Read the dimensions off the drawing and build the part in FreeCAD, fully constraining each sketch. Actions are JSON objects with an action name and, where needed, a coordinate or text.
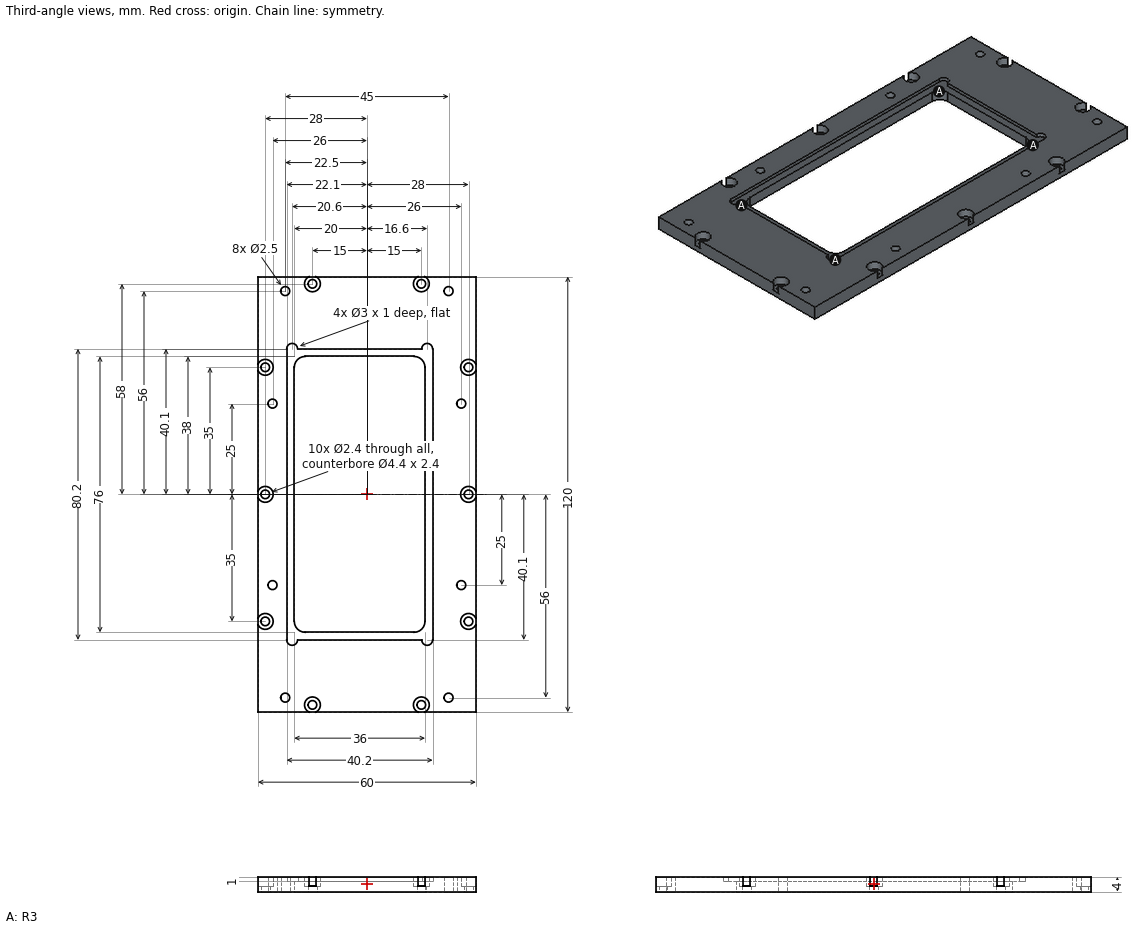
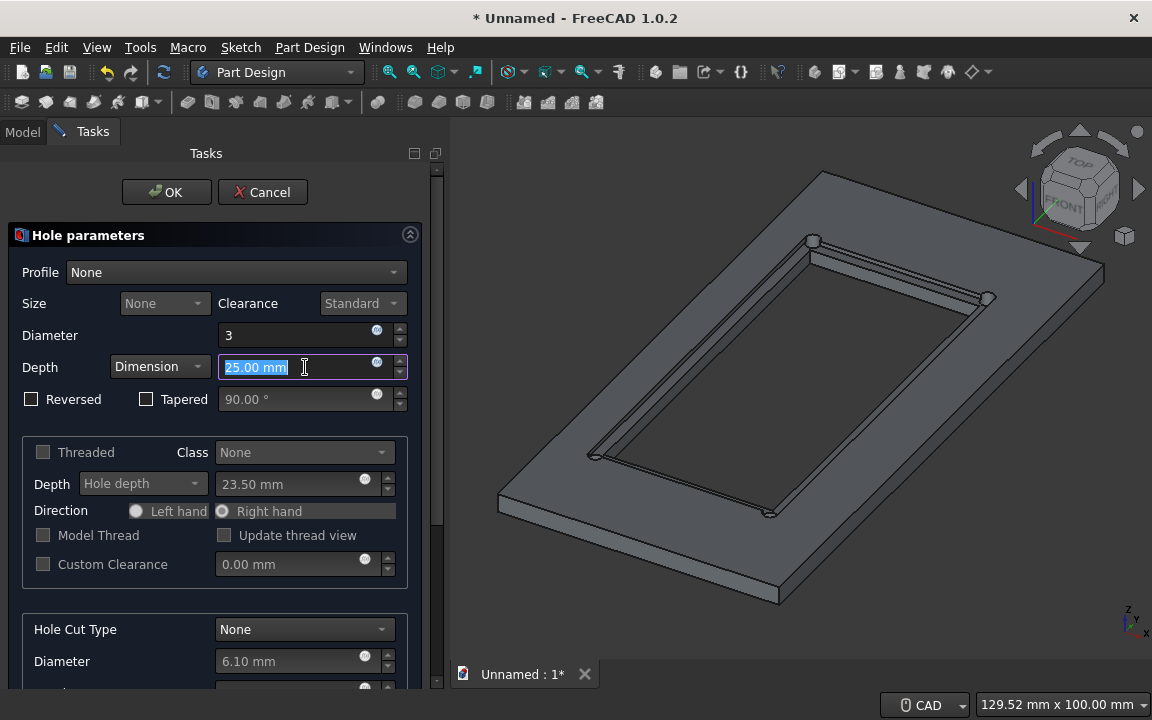
{"action": "type", "text": "1"}
{"action": "key", "text": "Tab"}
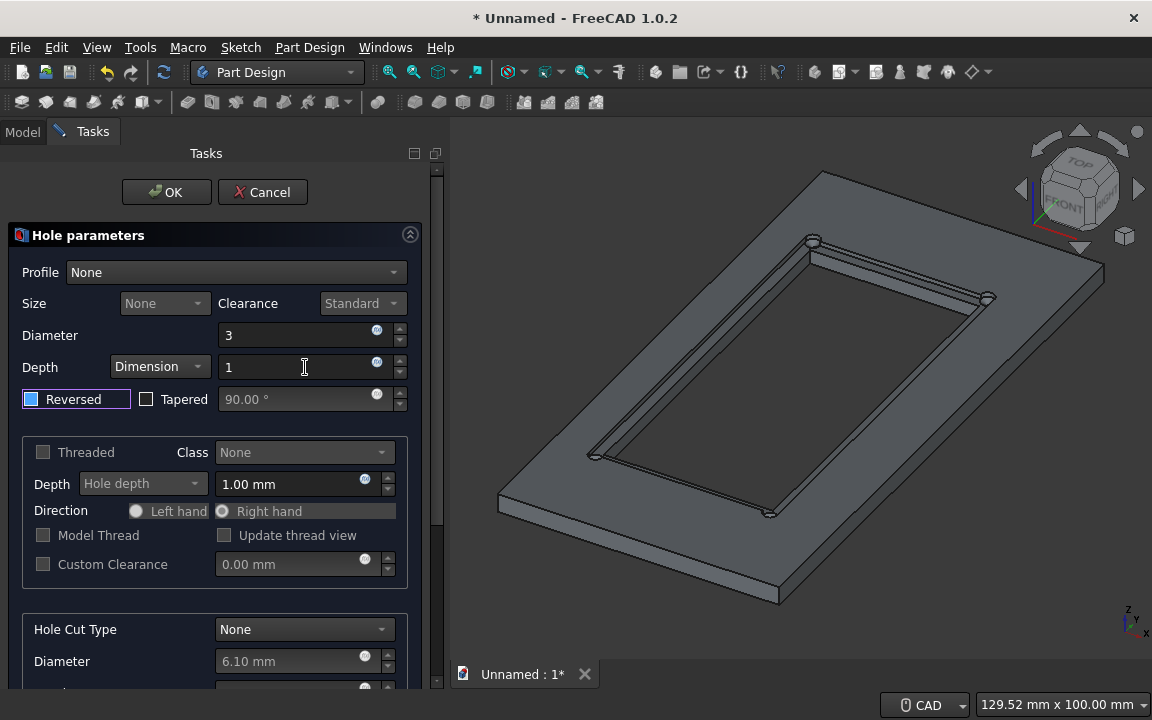
{"action": "scroll", "coordinate": [437, 426], "scroll_direction": "down", "scroll_amount": 4}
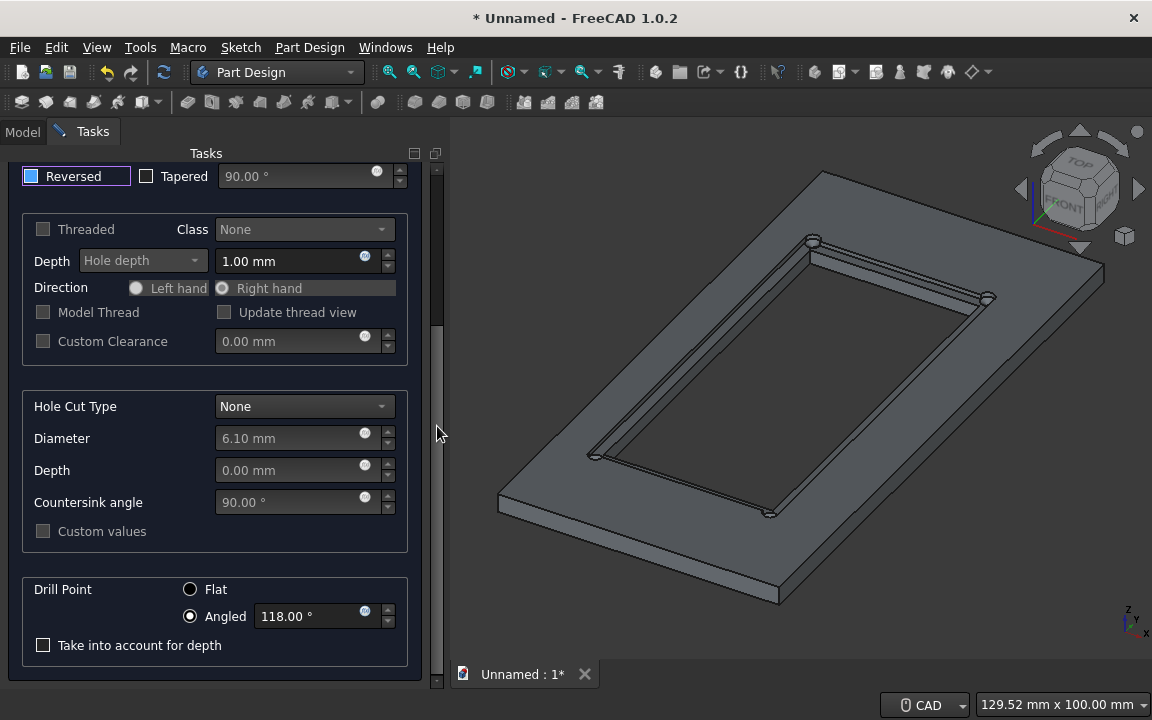
{"action": "left_click", "coordinate": [191, 589]}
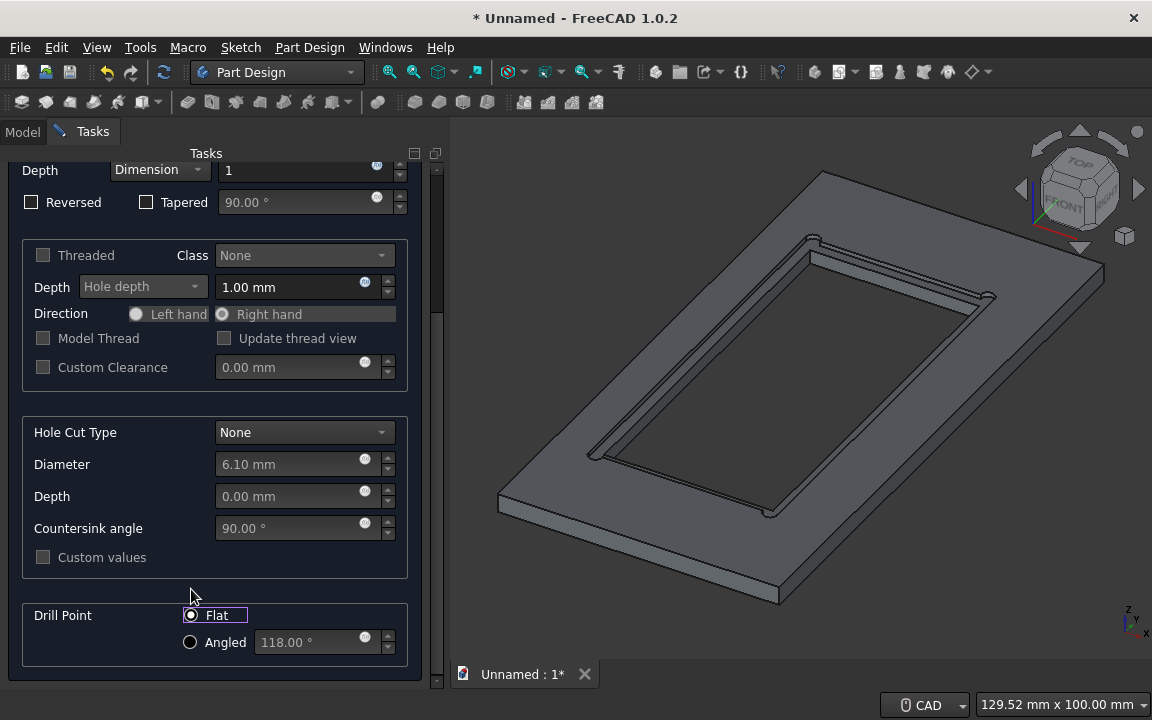
{"action": "scroll", "coordinate": [437, 426], "scroll_direction": "up", "scroll_amount": 5}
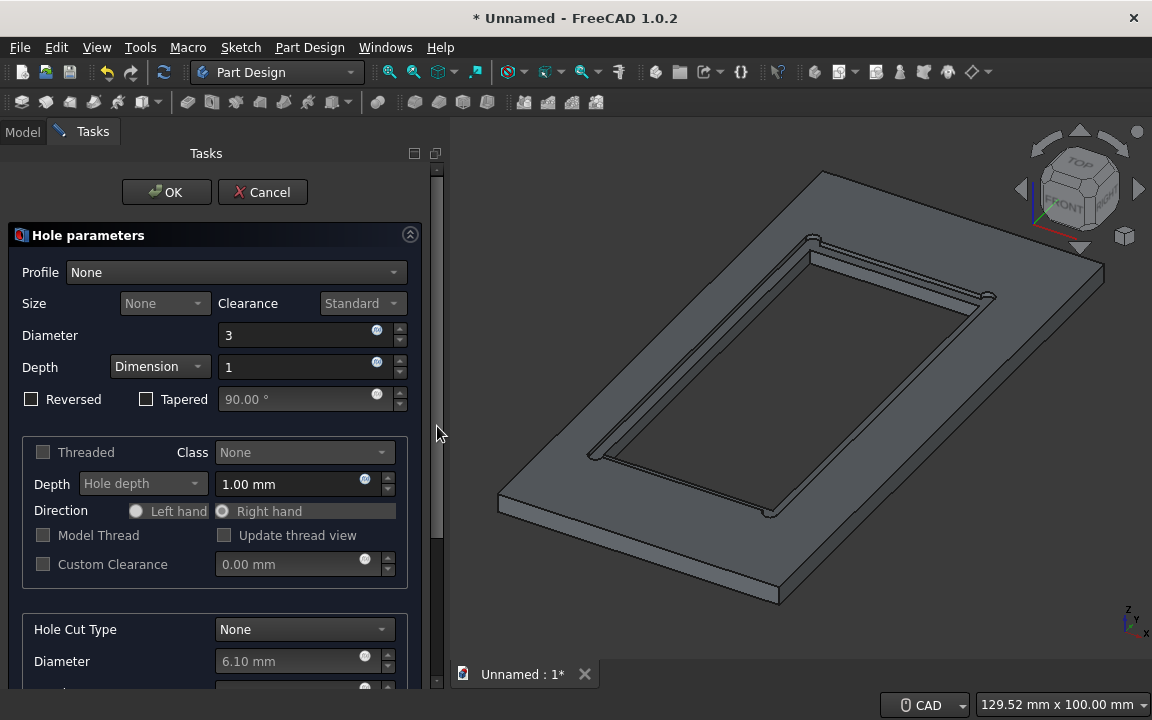
{"action": "left_click", "coordinate": [167, 192]}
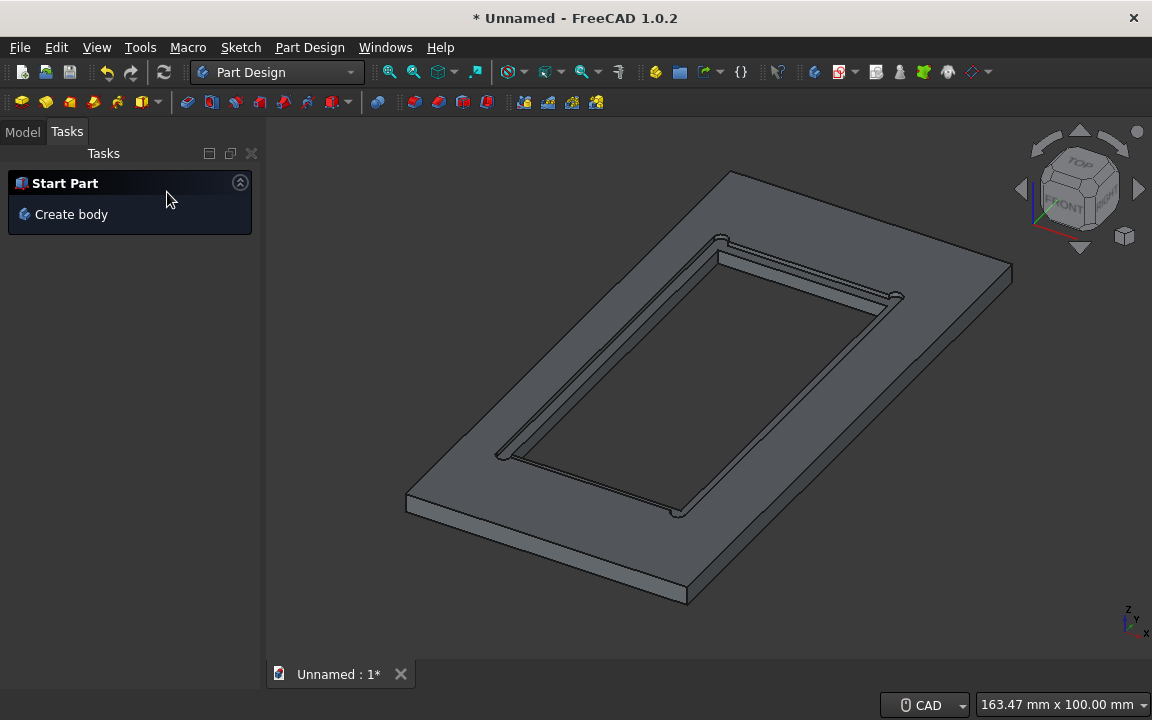
{"action": "scroll", "coordinate": [512, 460], "scroll_direction": "up", "scroll_amount": 5}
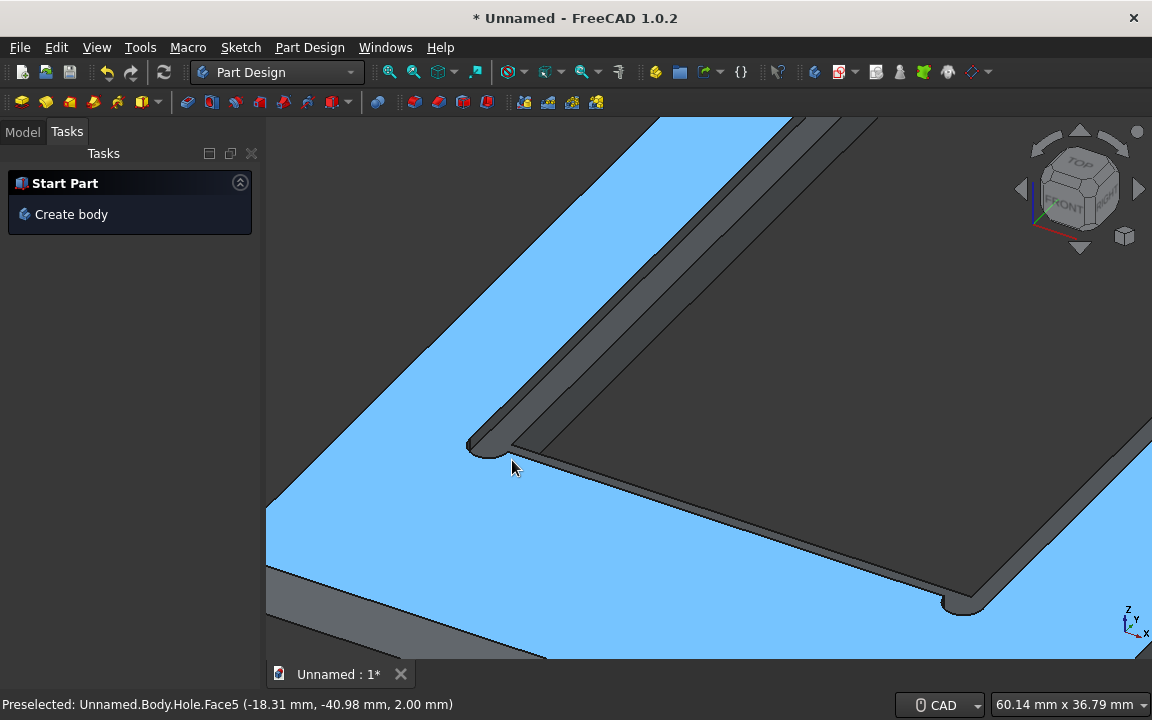
{"action": "key", "text": "v f"}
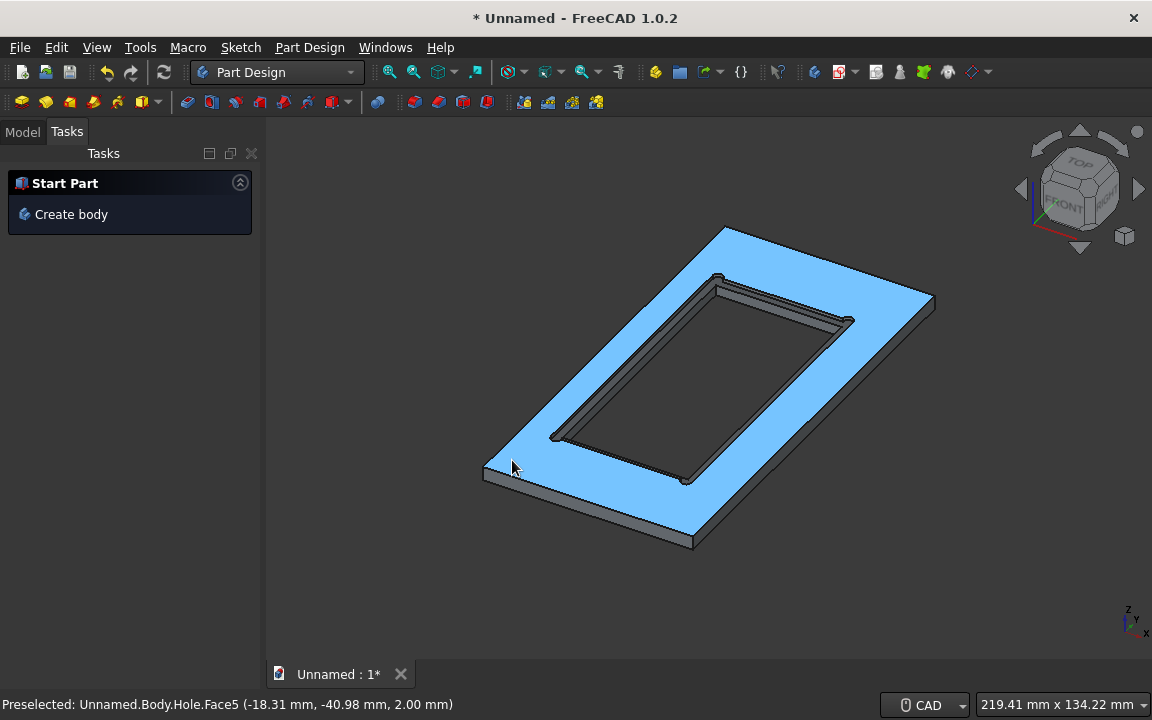
{"action": "key", "text": "0"}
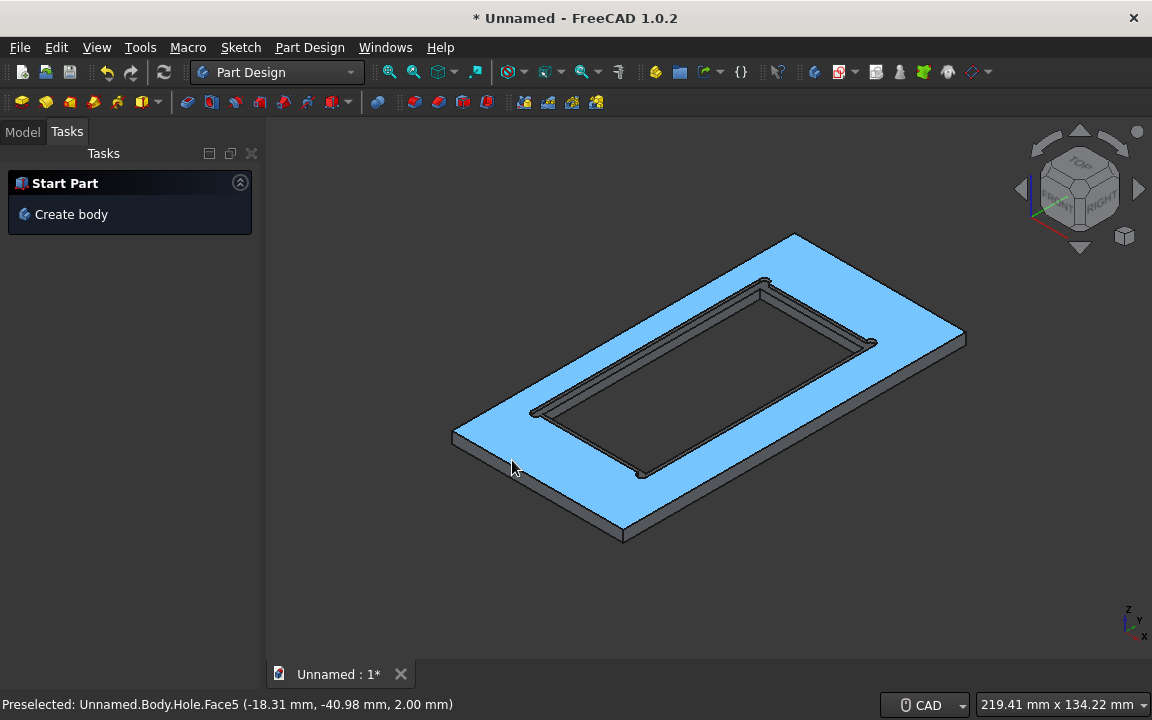
{"action": "scroll", "coordinate": [543, 418], "scroll_direction": "up", "scroll_amount": 6}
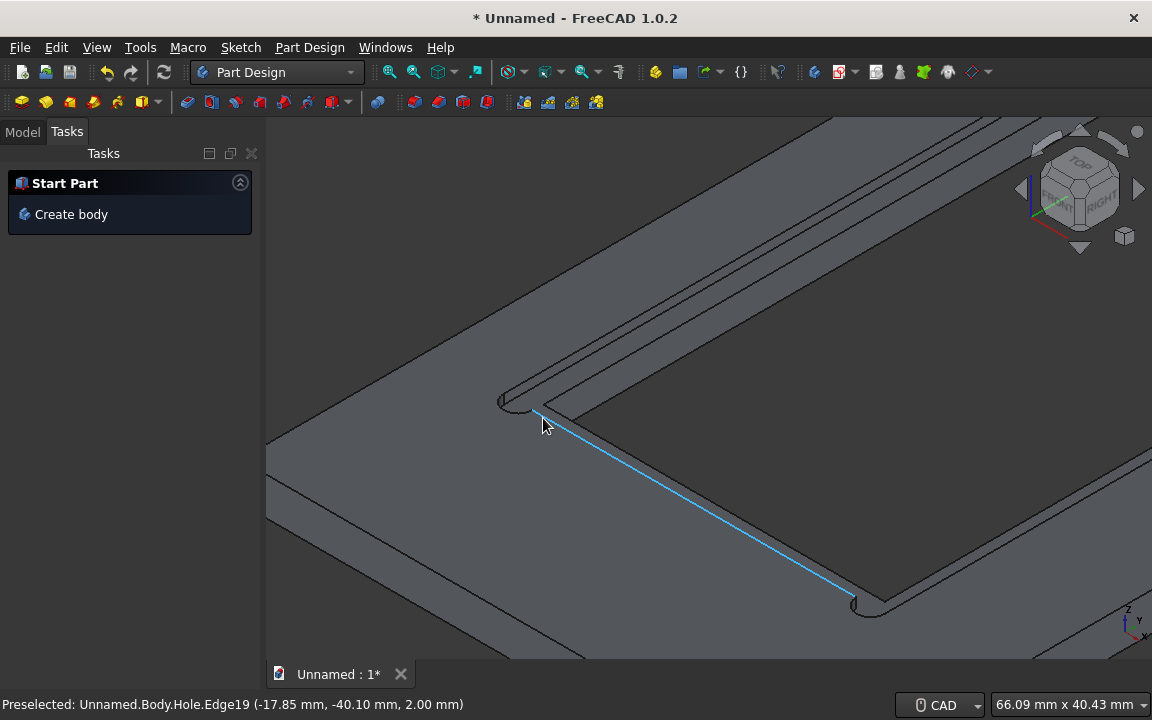
{"action": "left_click", "coordinate": [390, 72]}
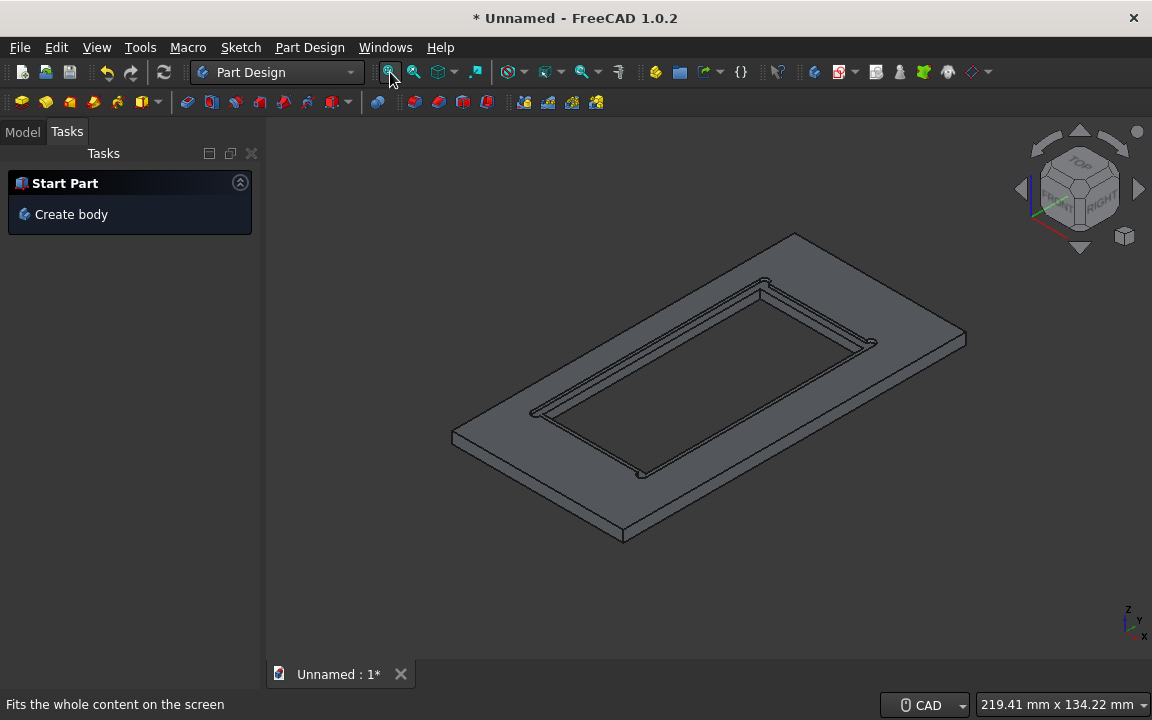
{"action": "key", "text": "2"}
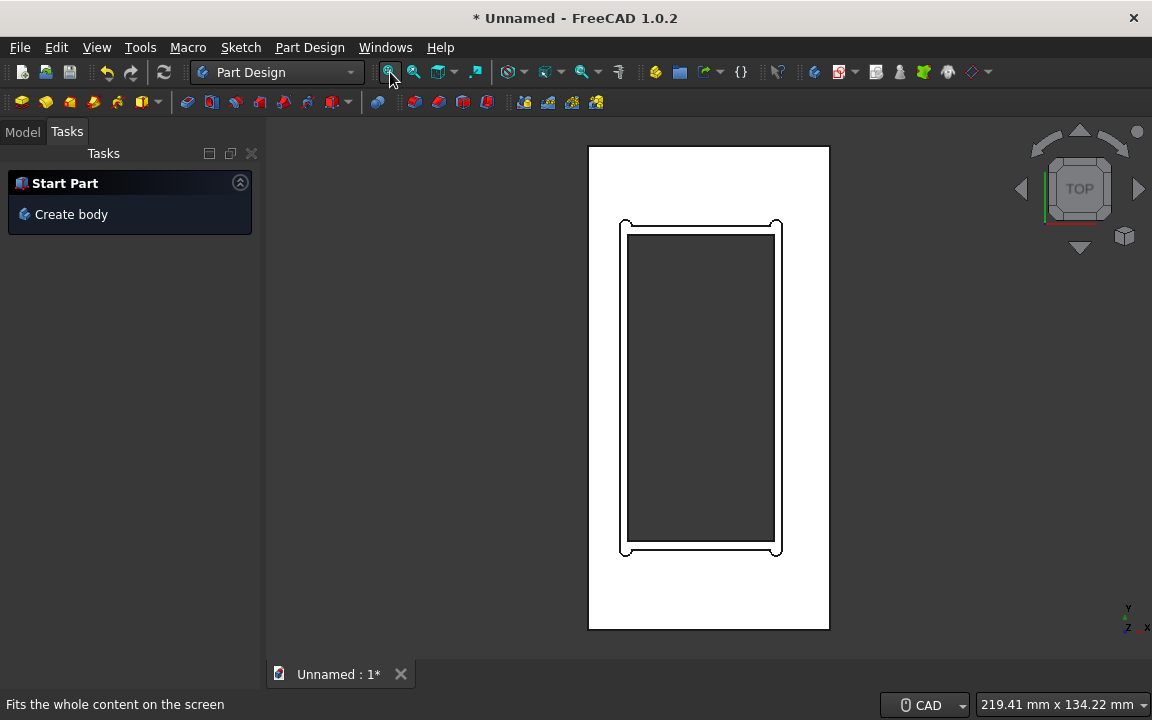
{"action": "scroll", "coordinate": [628, 540], "scroll_direction": "up", "scroll_amount": 6}